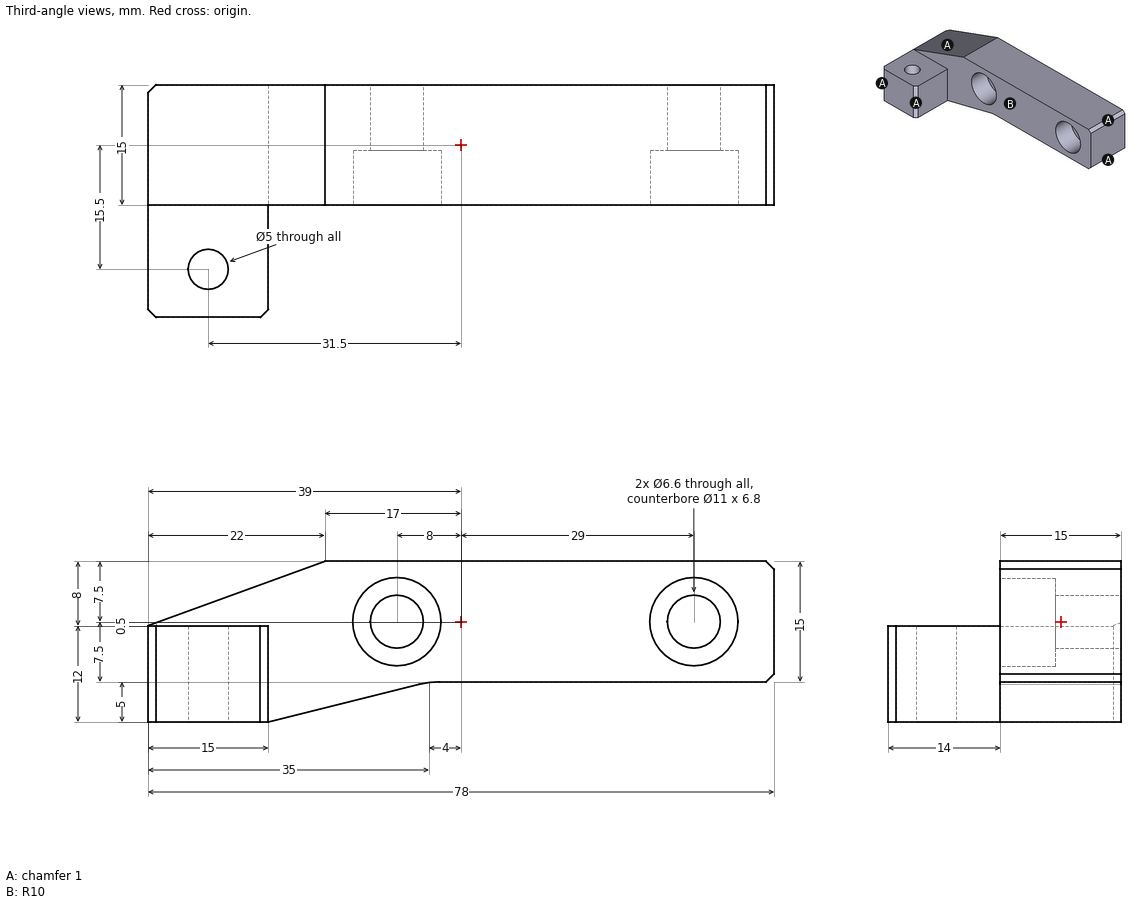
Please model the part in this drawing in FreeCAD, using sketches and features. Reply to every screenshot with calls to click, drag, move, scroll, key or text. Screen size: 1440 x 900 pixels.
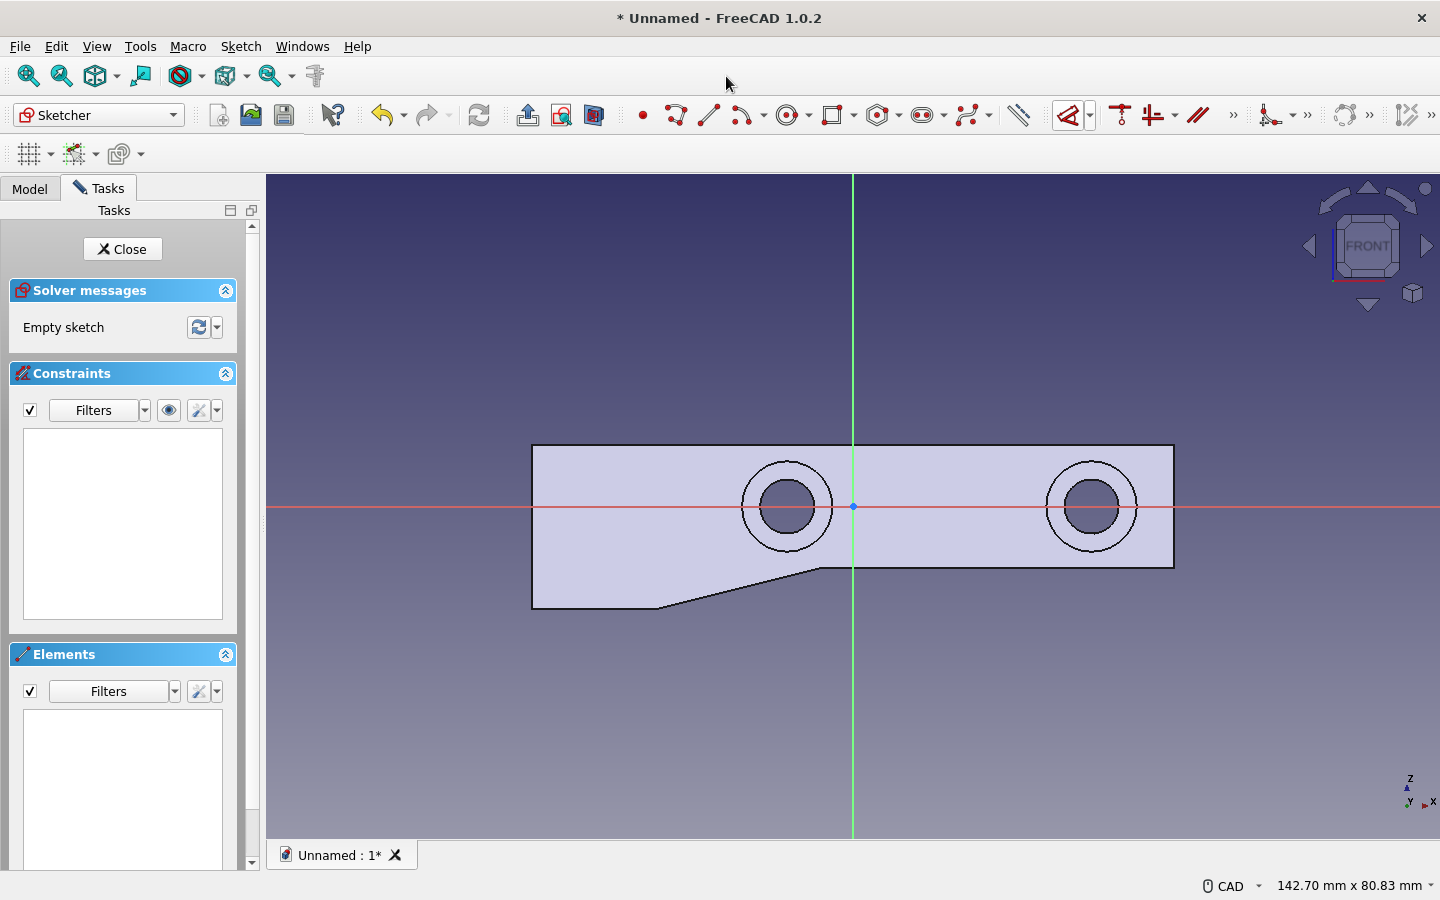
scroll(531, 577, up, 7)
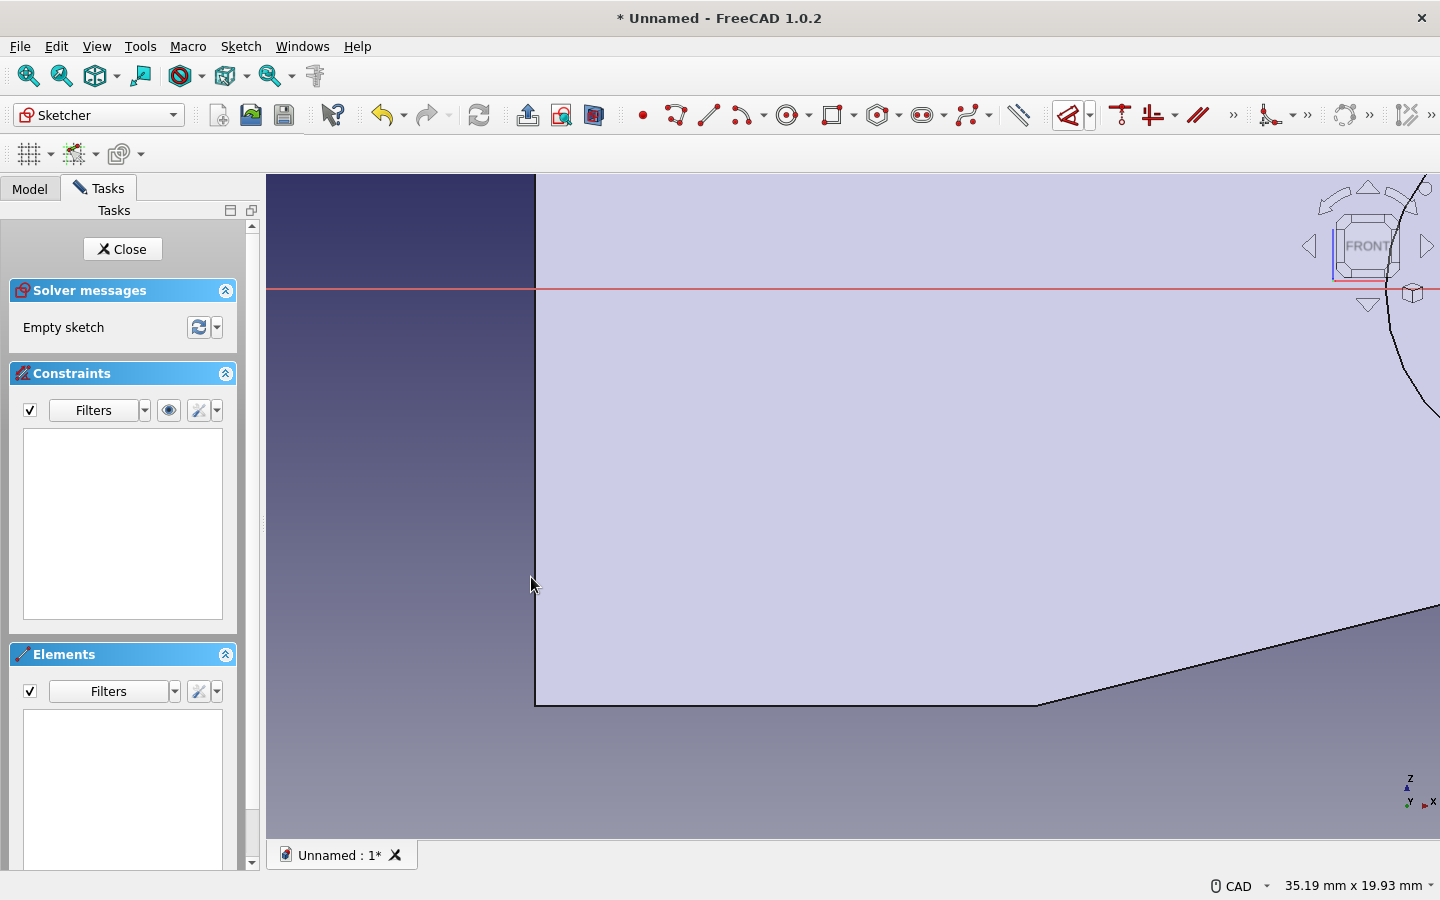
click(832, 116)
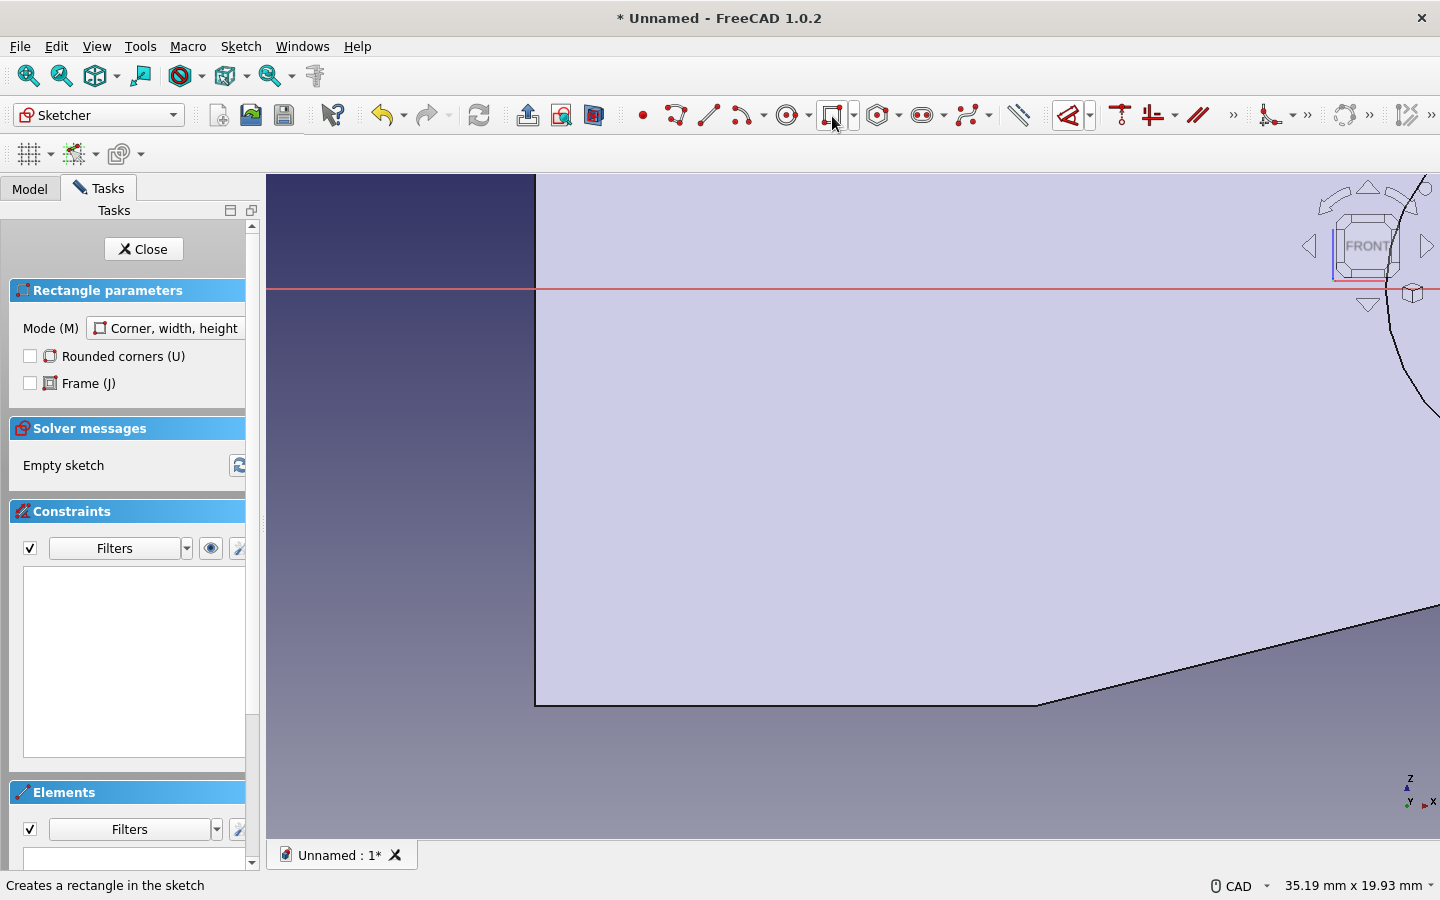
click(535, 306)
move(1035, 706)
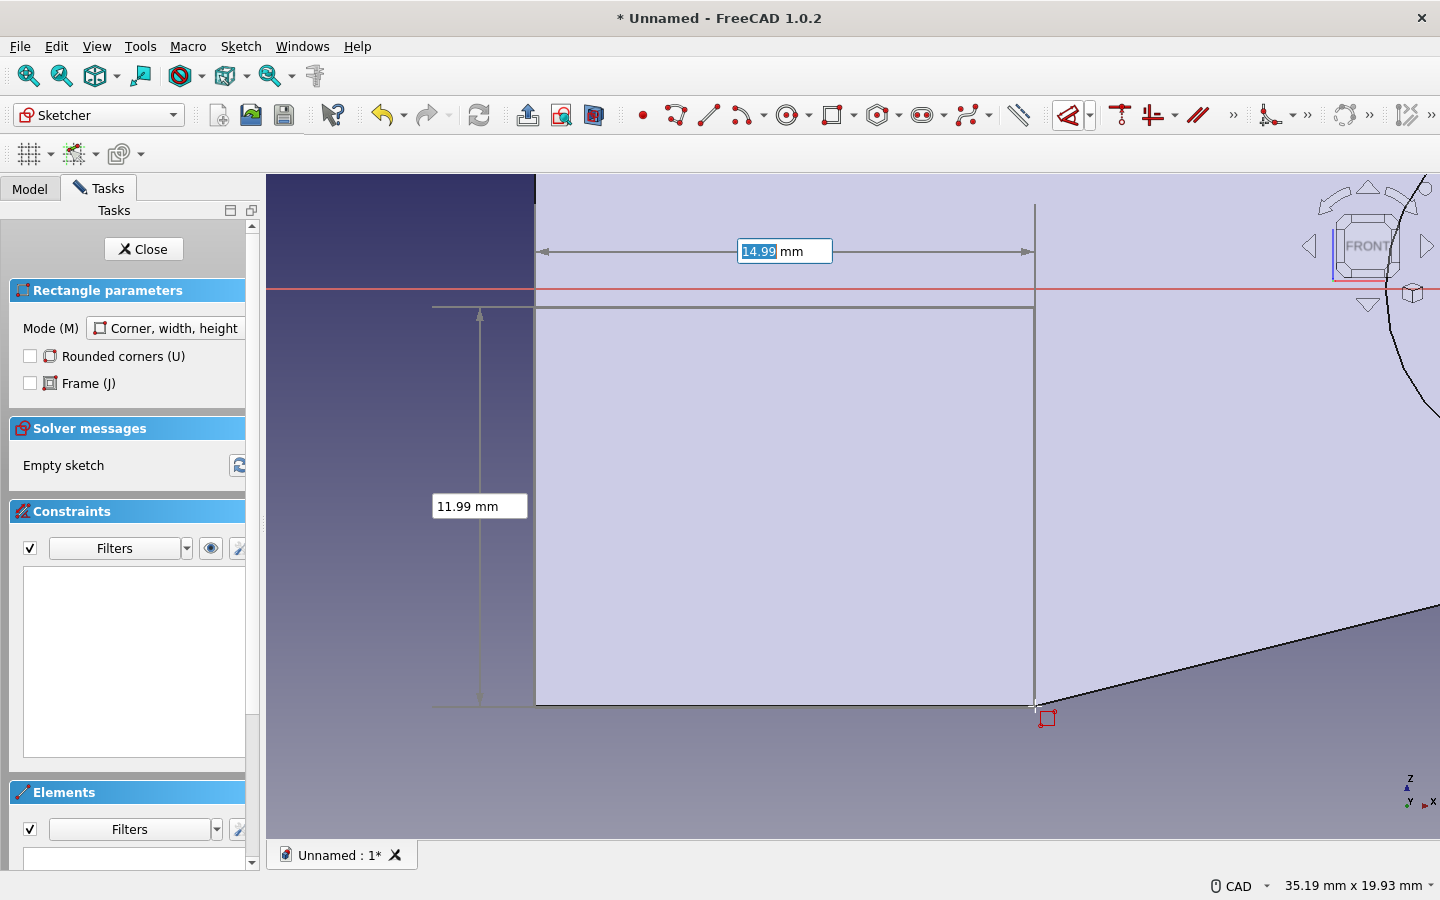
text(15)
key(Tab)
text(12)
key(Return)
key(Escape)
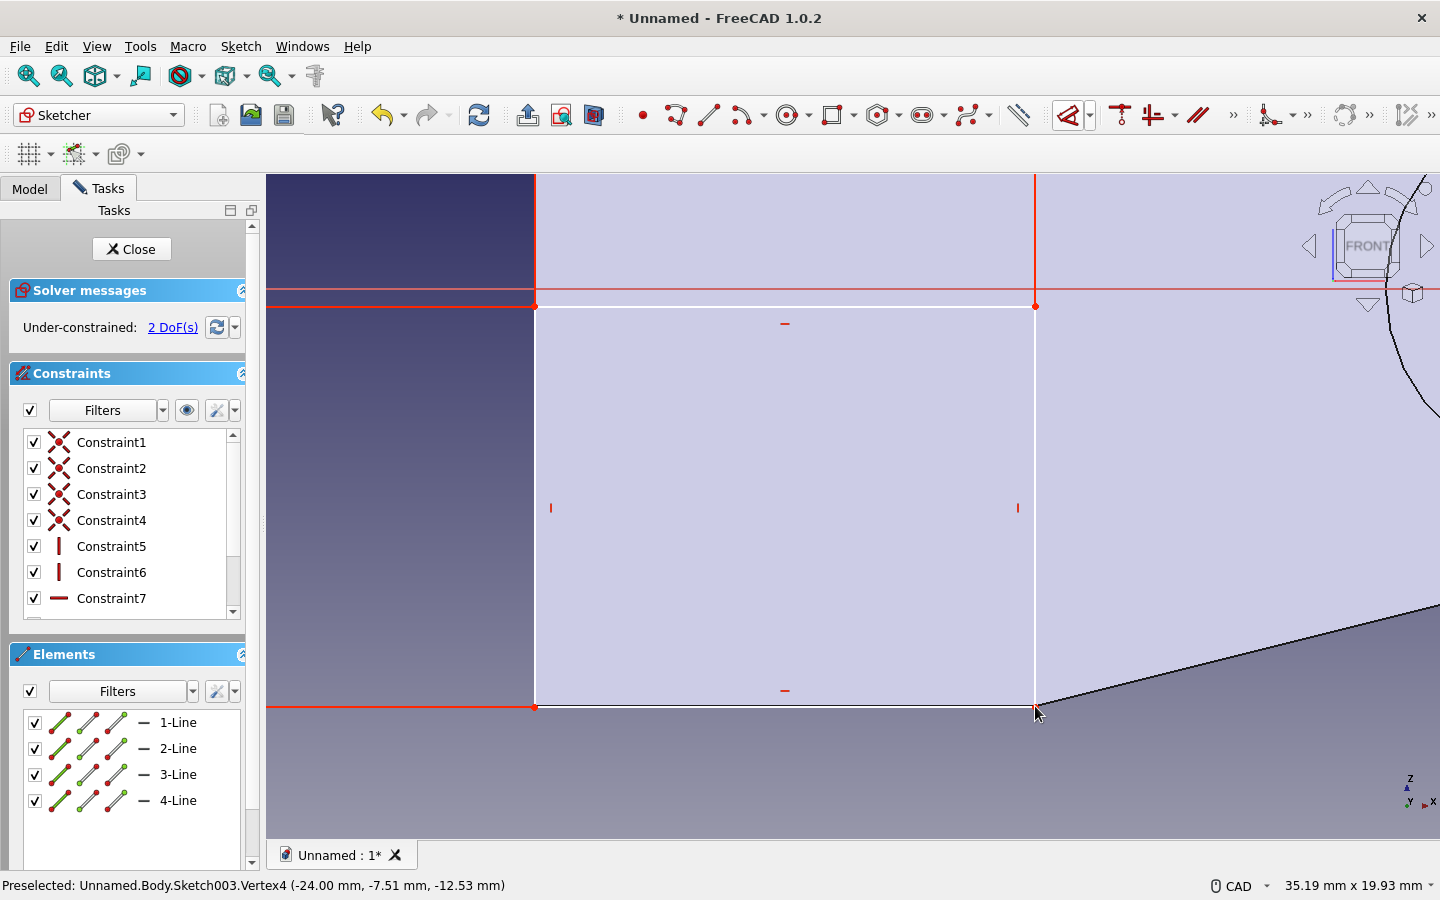
click(535, 307)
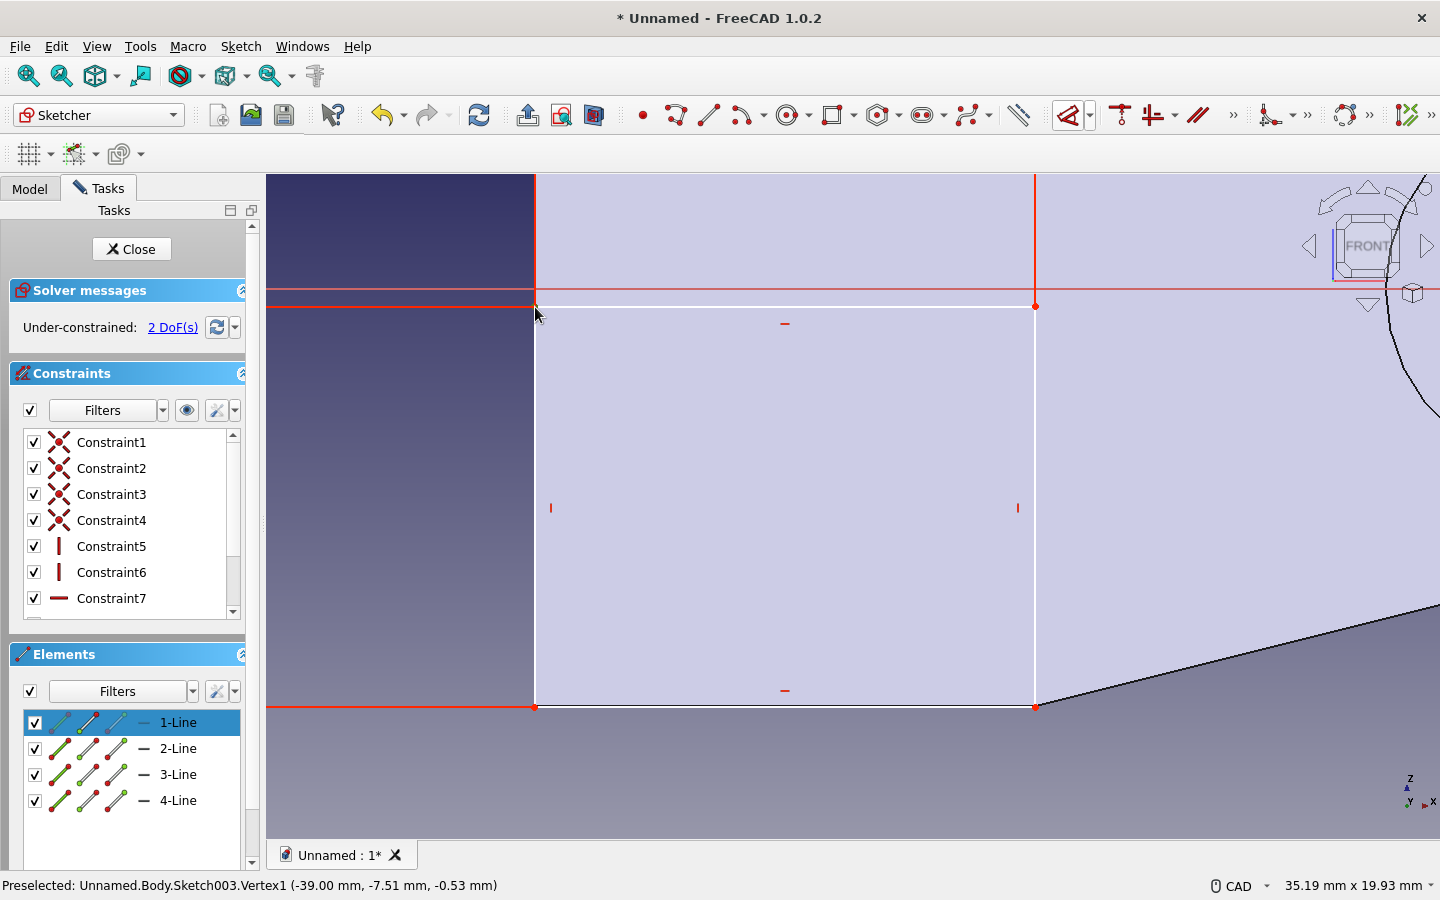
key(l)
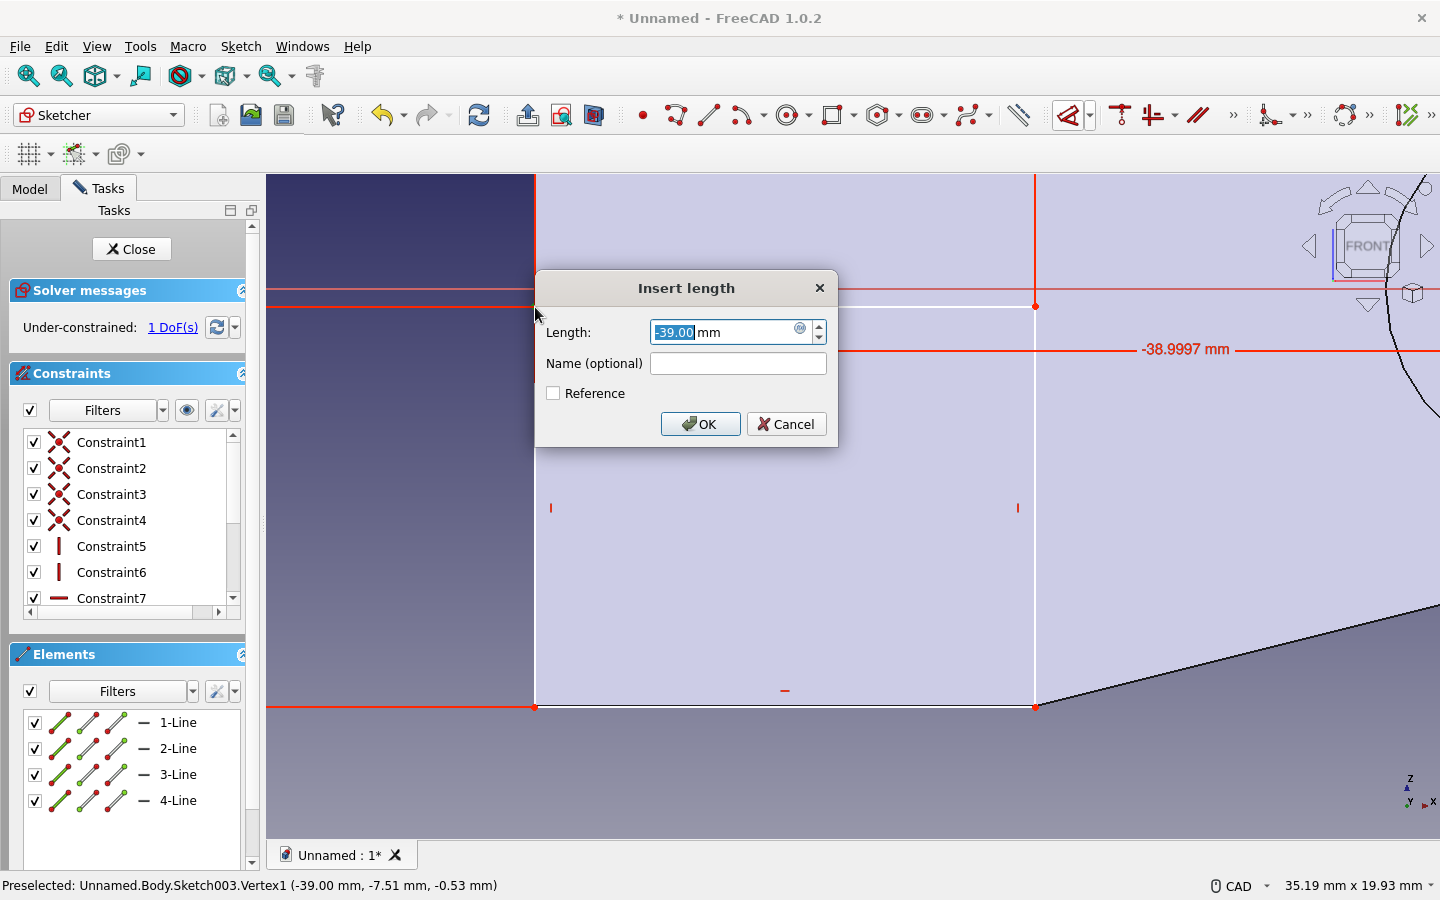
text(-39)
key(Return)